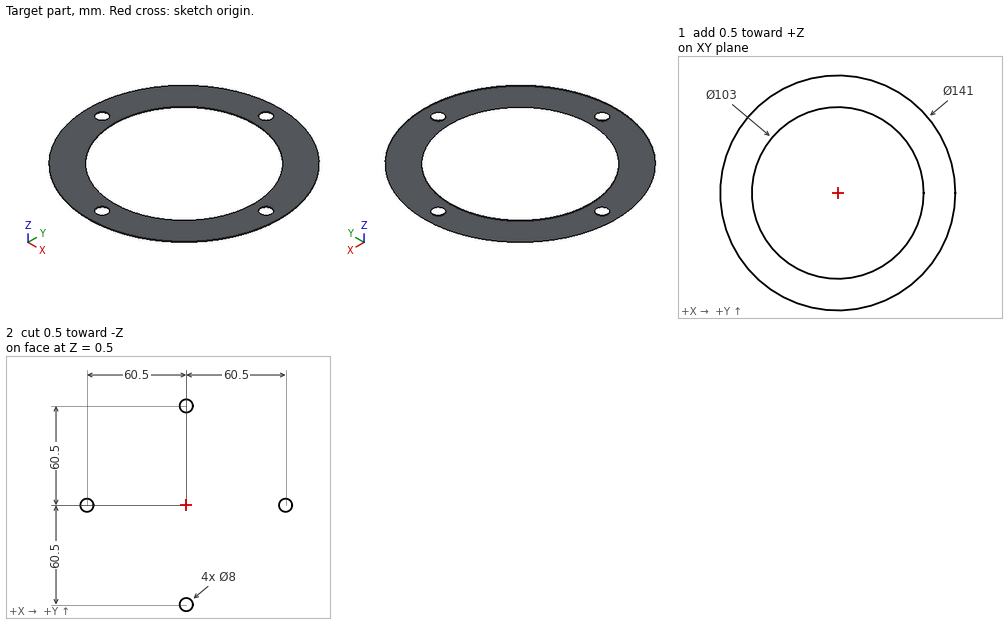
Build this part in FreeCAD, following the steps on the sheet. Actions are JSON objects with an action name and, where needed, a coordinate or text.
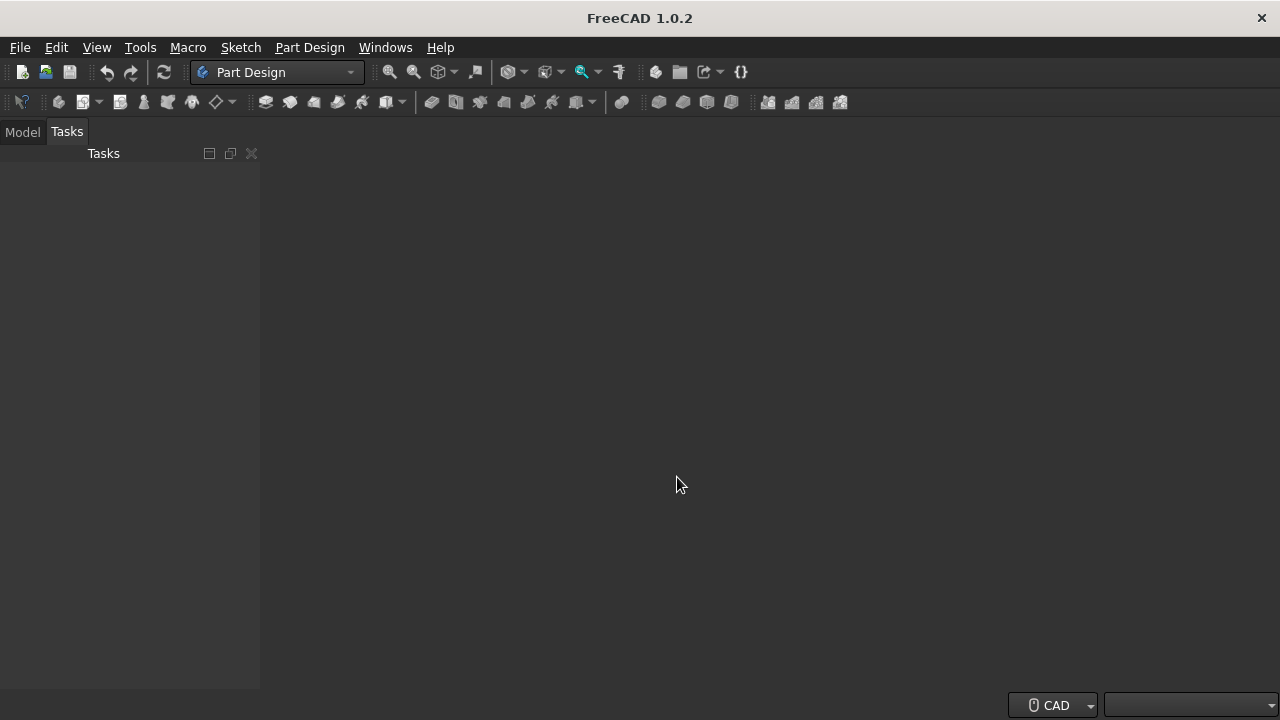
{"action": "left_click", "coordinate": [22, 72]}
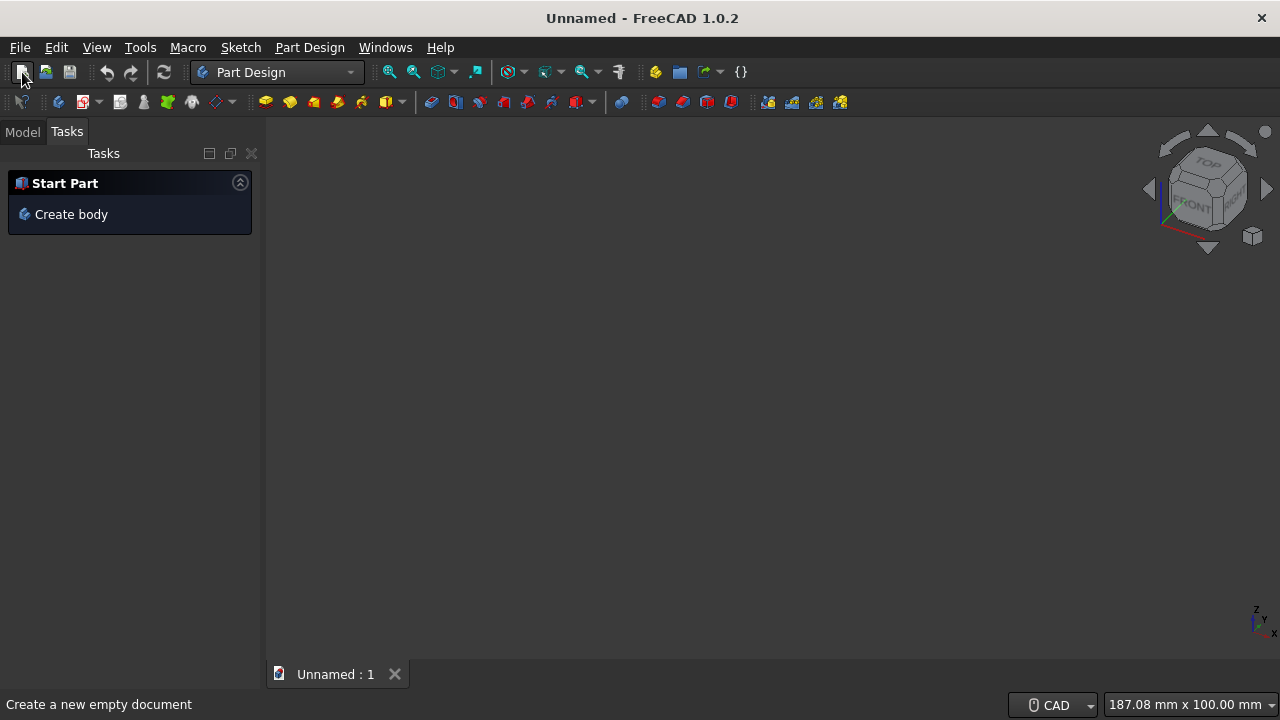
{"action": "left_click", "coordinate": [84, 102]}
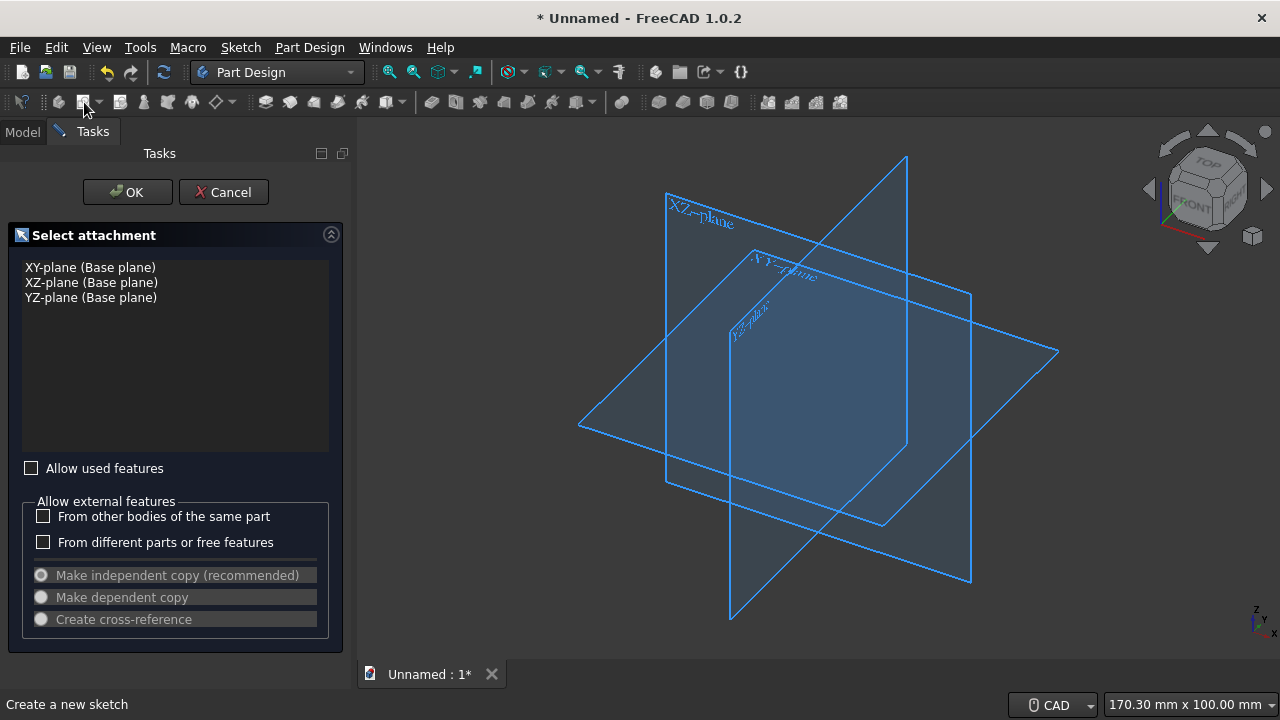
{"action": "left_click", "coordinate": [82, 268]}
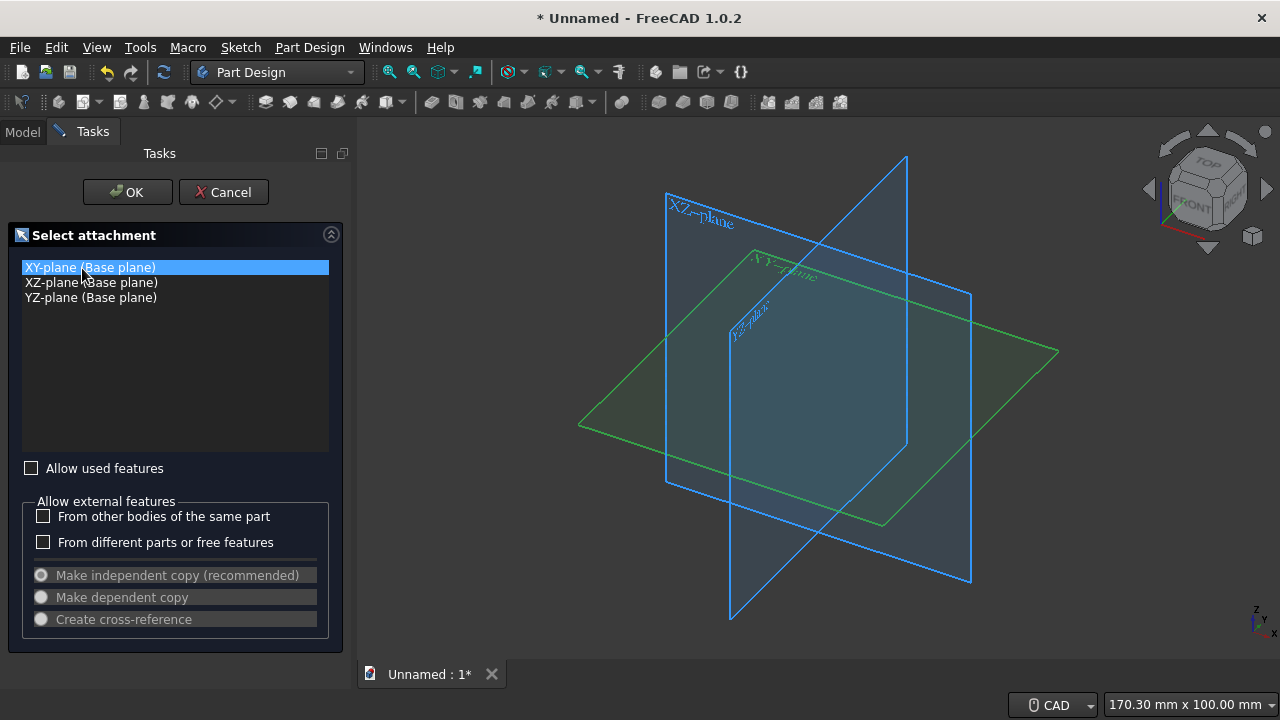
{"action": "left_click", "coordinate": [128, 192]}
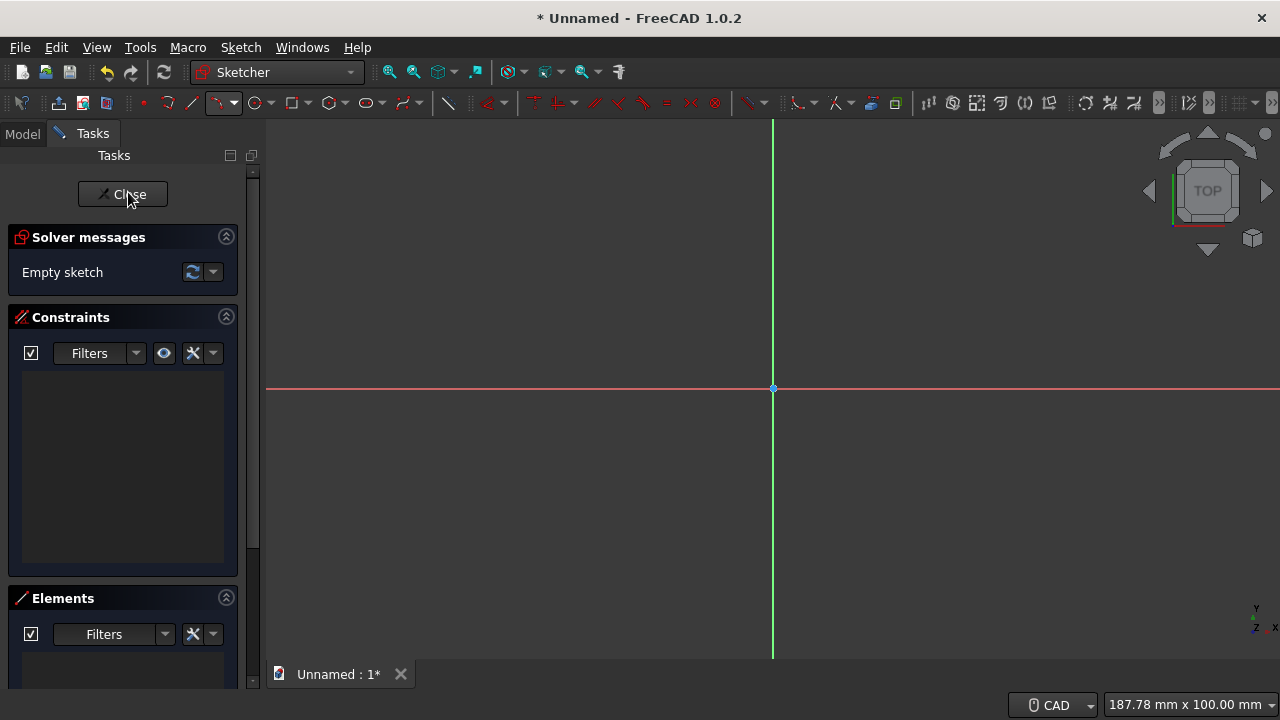
{"action": "scroll", "coordinate": [649, 389], "scroll_direction": "down", "scroll_amount": 4}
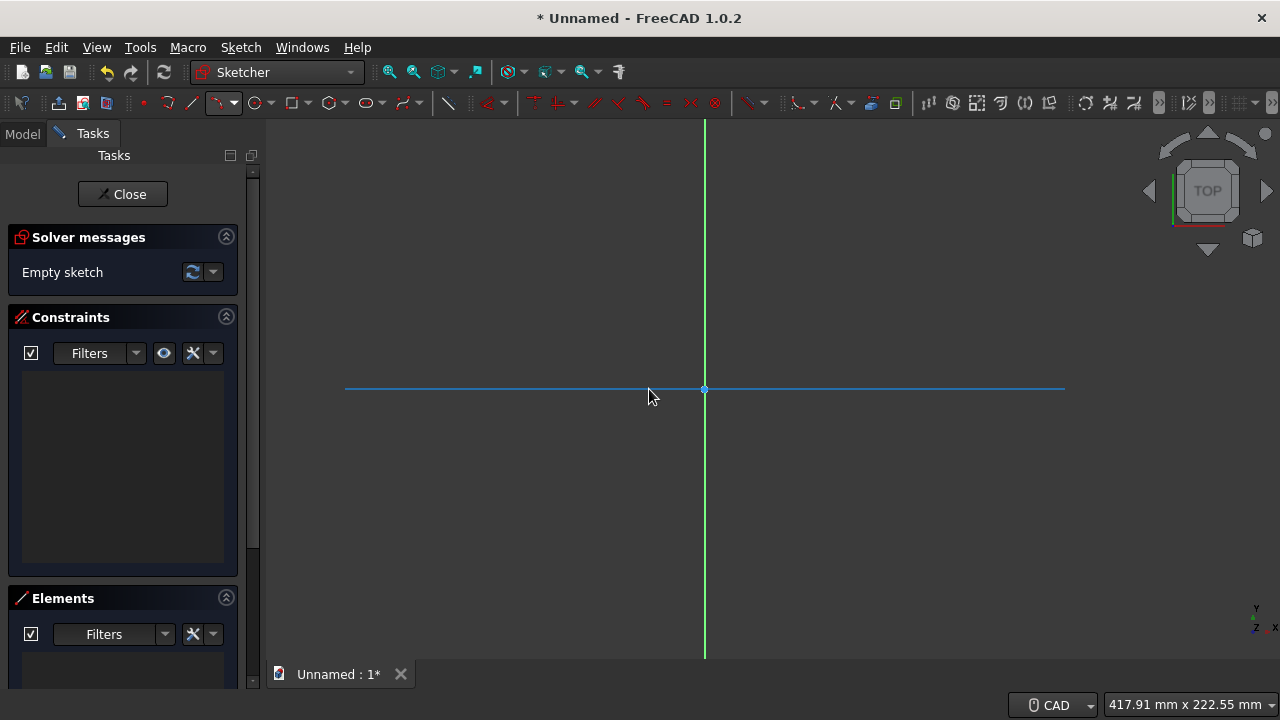
{"action": "left_click", "coordinate": [256, 104]}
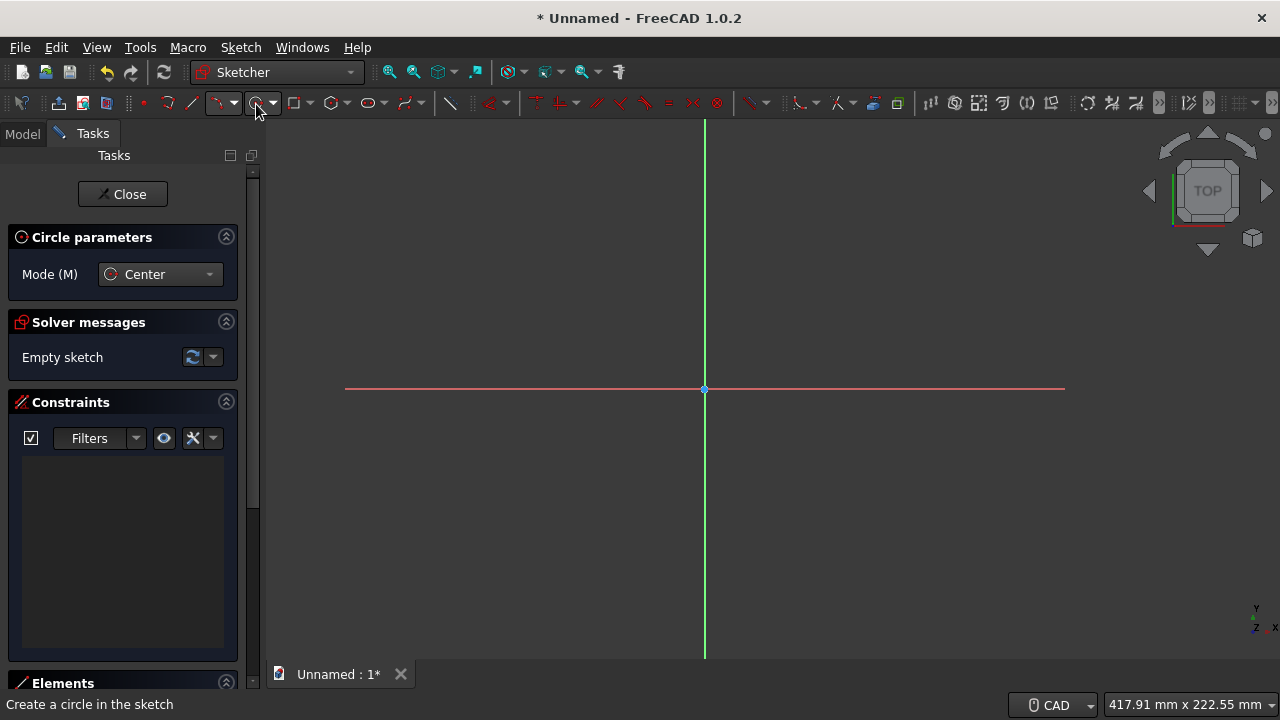
{"action": "left_click", "coordinate": [705, 389]}
{"action": "left_click", "coordinate": [826, 268]}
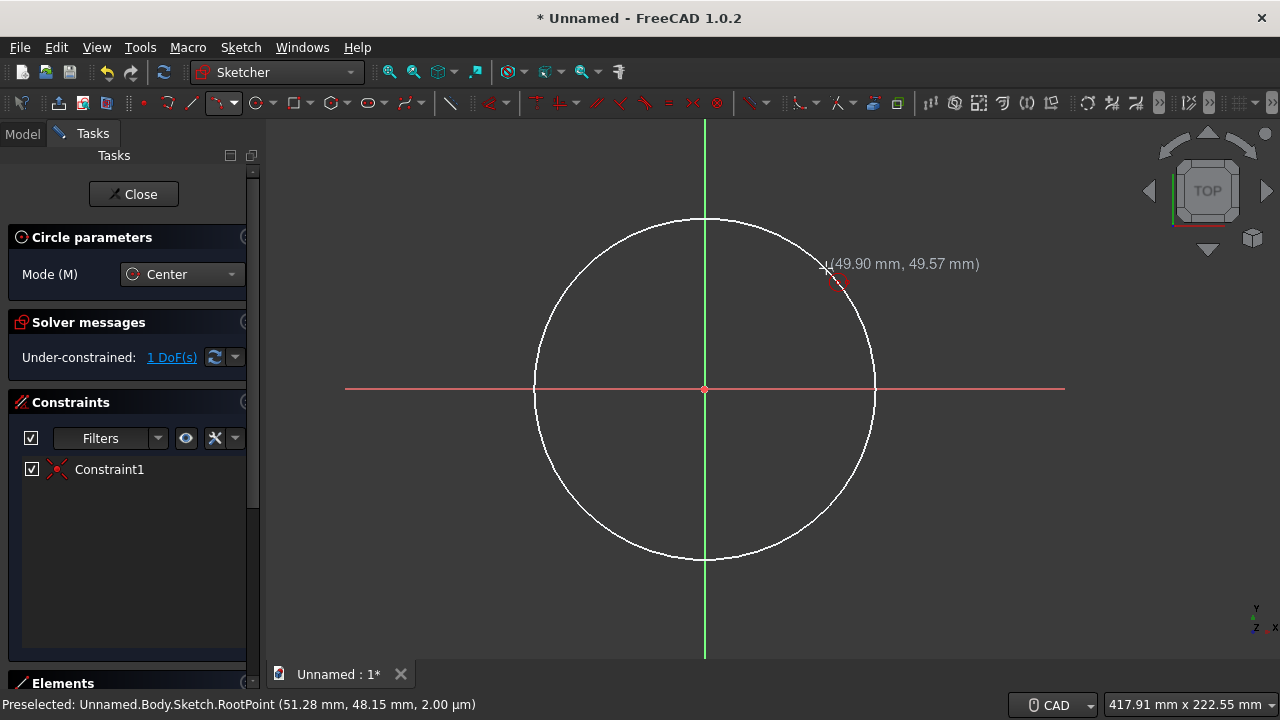
{"action": "left_click", "coordinate": [705, 389]}
{"action": "left_click", "coordinate": [793, 301]}
{"action": "key", "text": "Escape"}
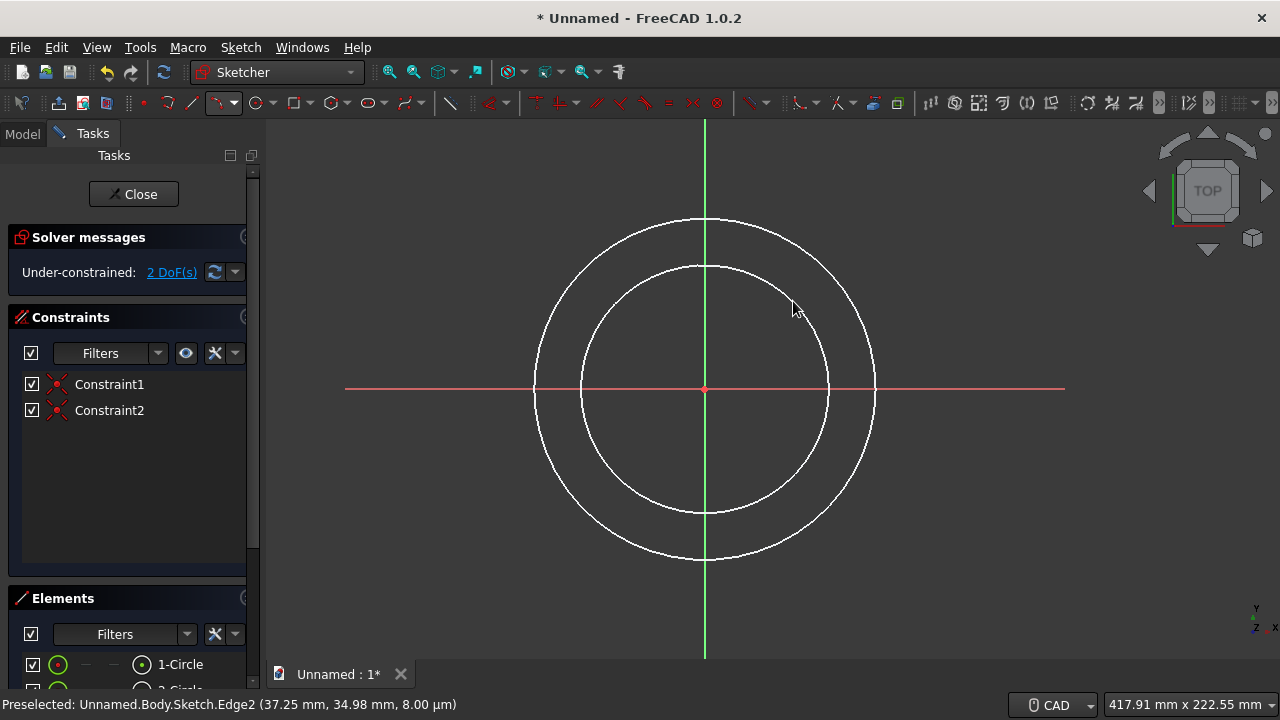
{"action": "left_click", "coordinate": [490, 104]}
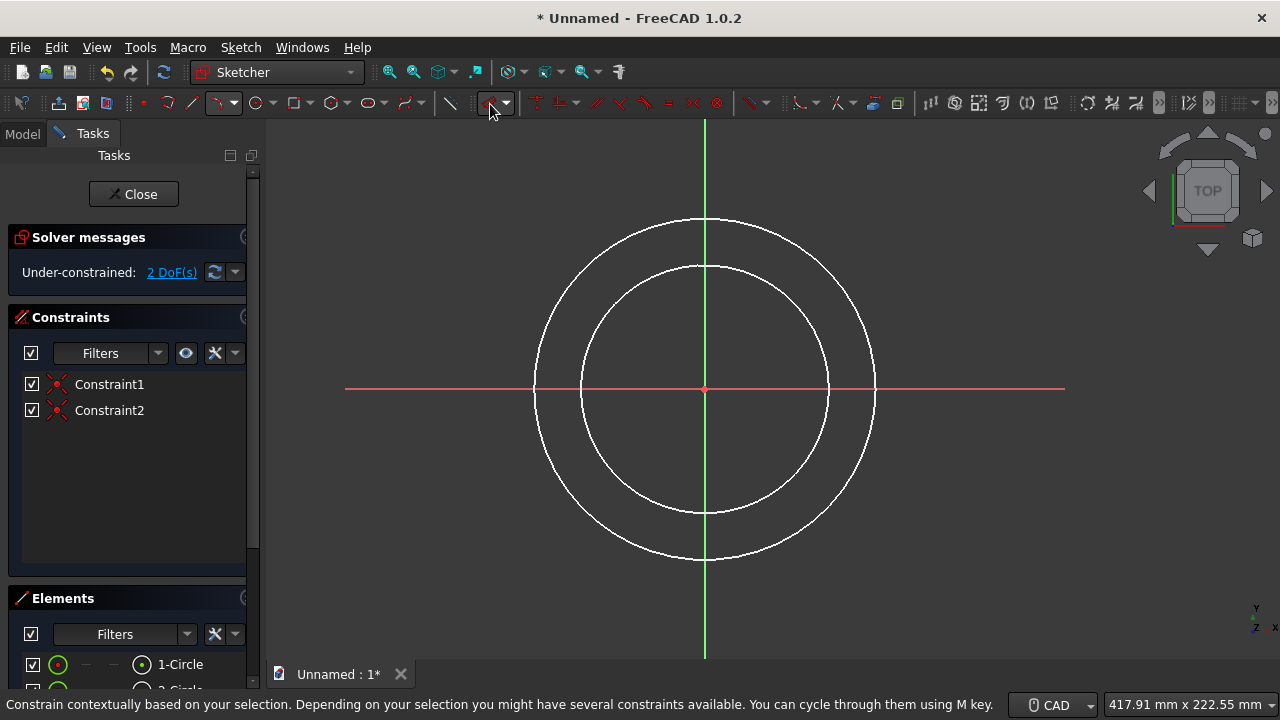
{"action": "left_click", "coordinate": [825, 268]}
{"action": "left_click", "coordinate": [848, 245]}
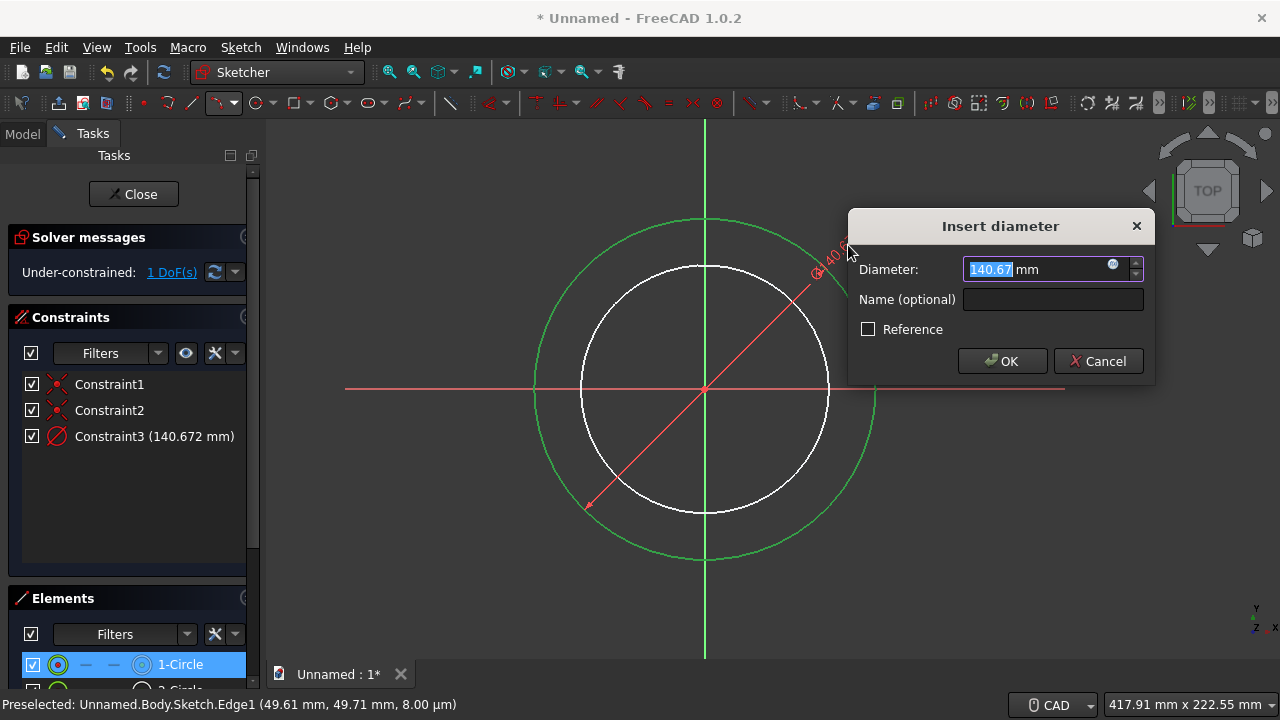
{"action": "type", "text": "141"}
{"action": "key", "text": "Return"}